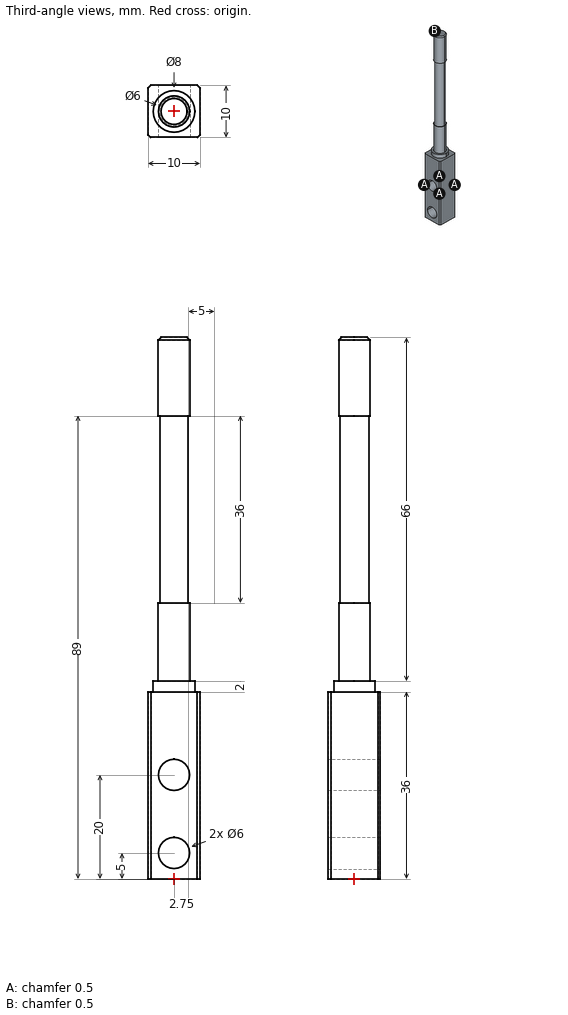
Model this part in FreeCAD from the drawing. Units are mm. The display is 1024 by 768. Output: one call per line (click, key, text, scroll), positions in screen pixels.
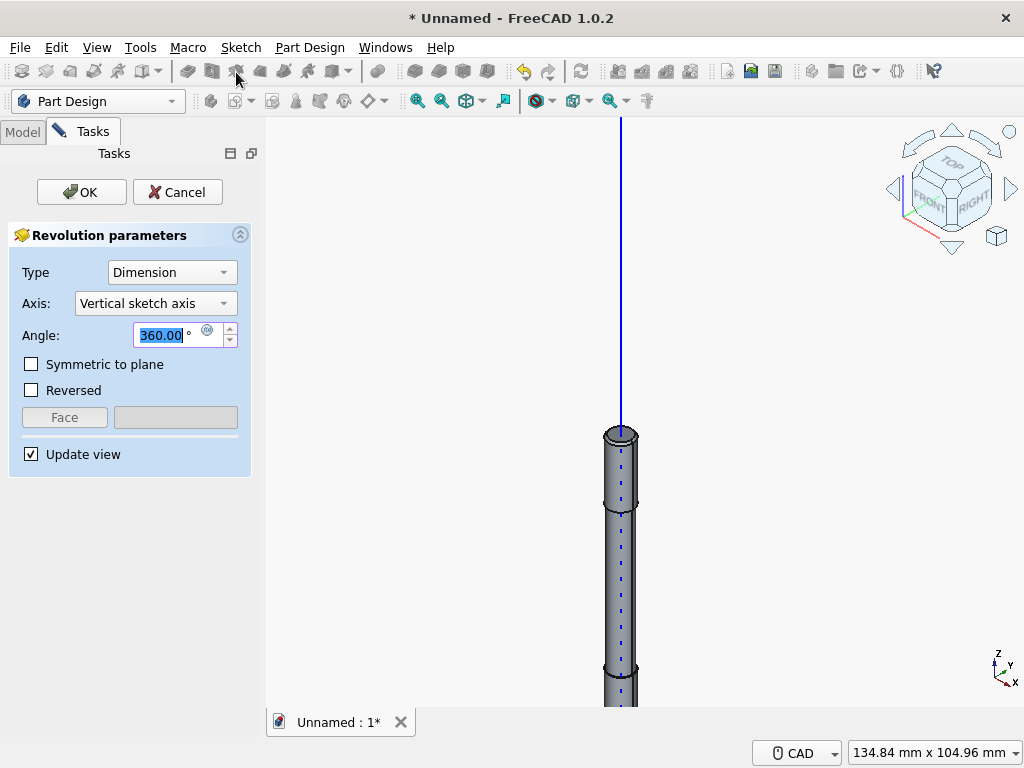
click(82, 192)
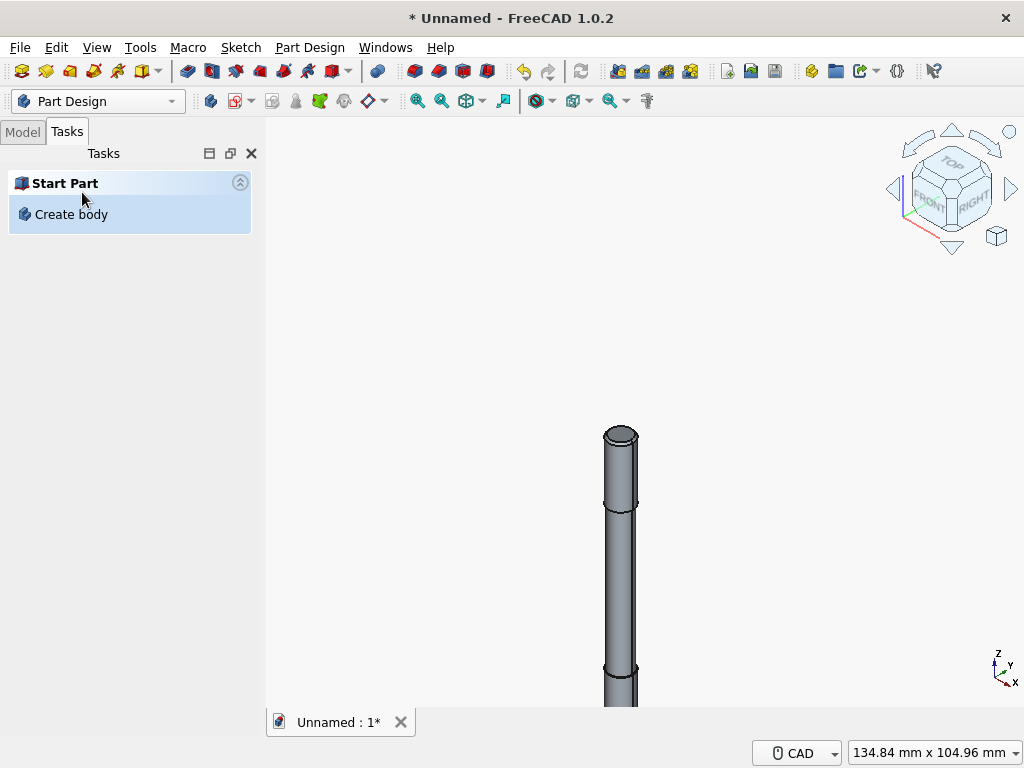
key(v)
key(f)